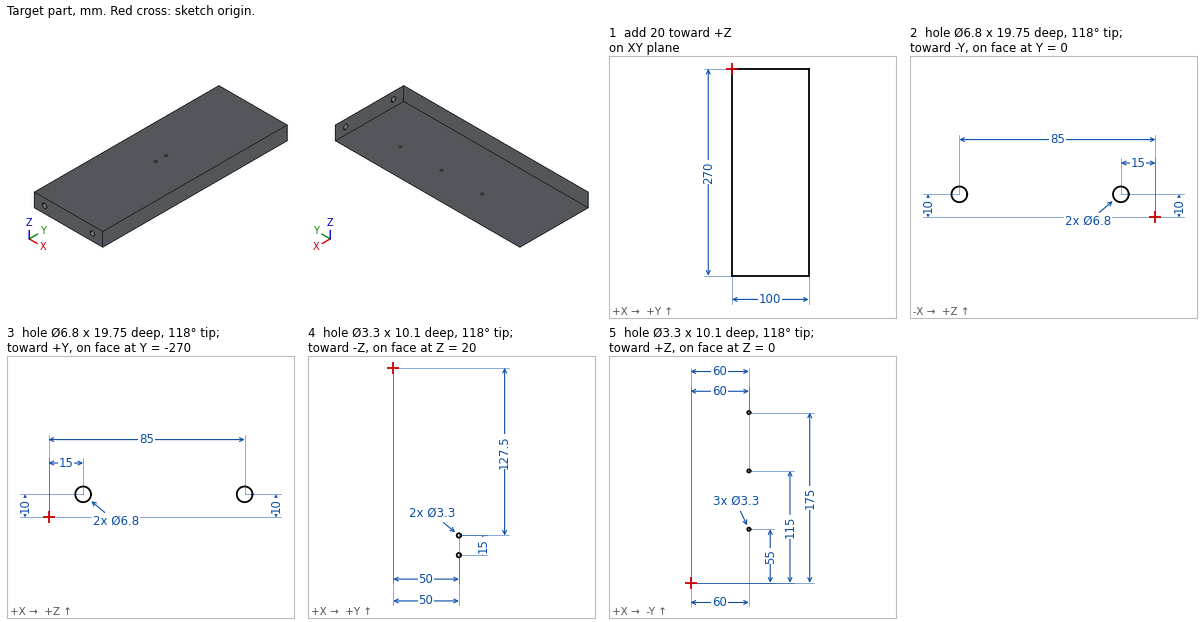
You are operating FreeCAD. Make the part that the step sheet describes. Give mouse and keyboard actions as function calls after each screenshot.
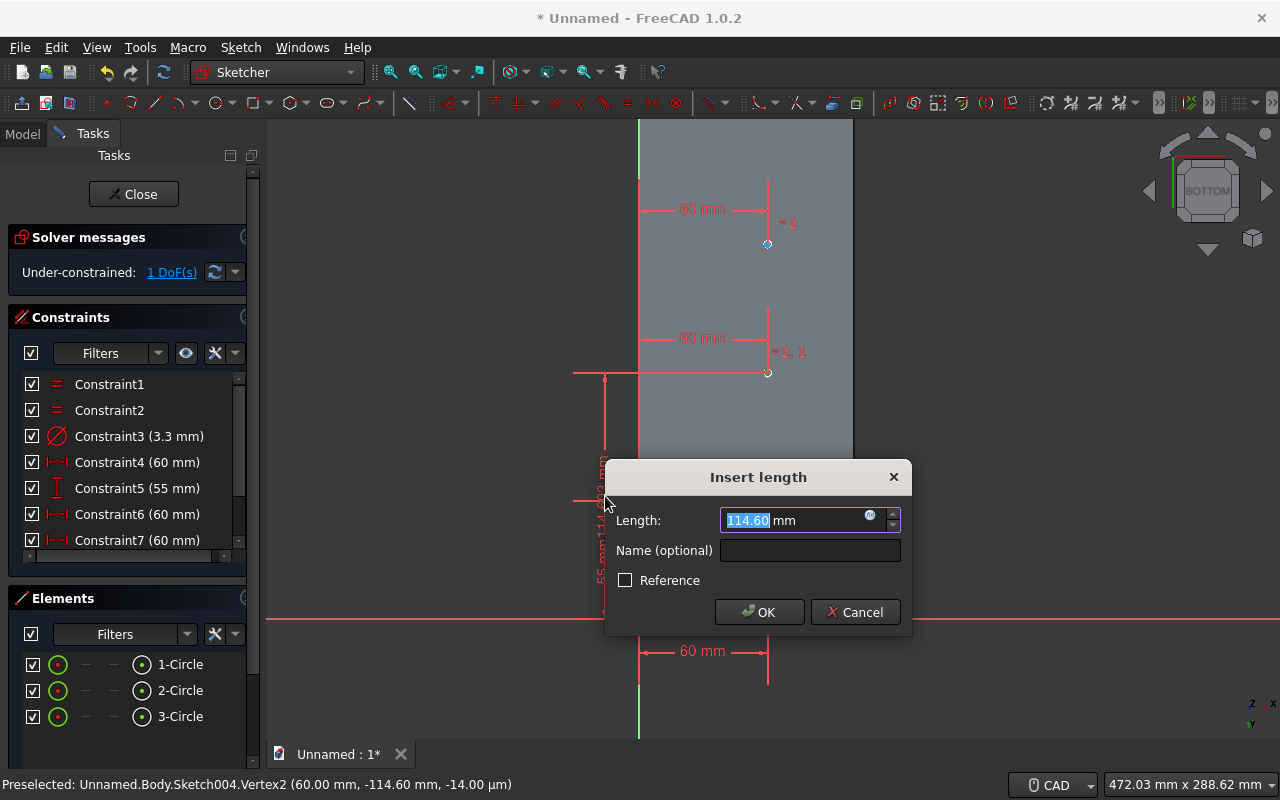
text(115)
key(Return)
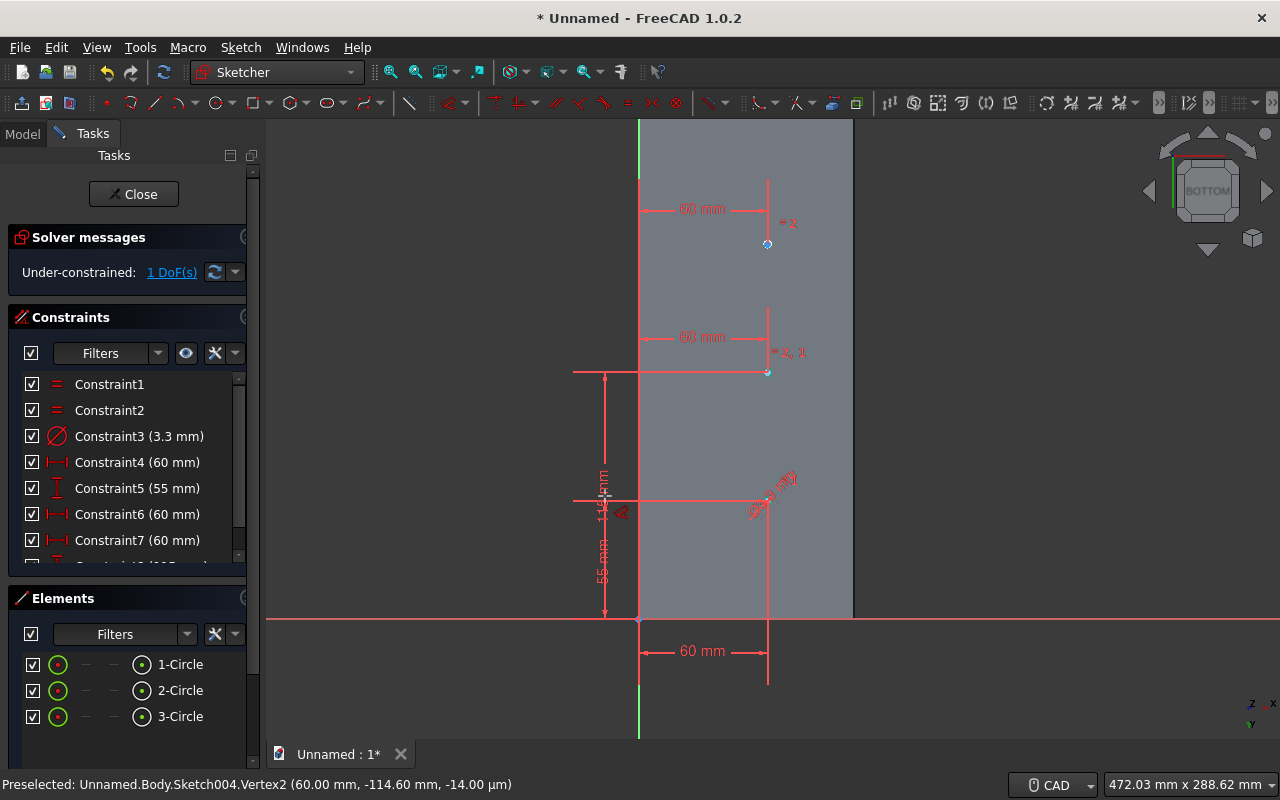
click(768, 244)
click(605, 432)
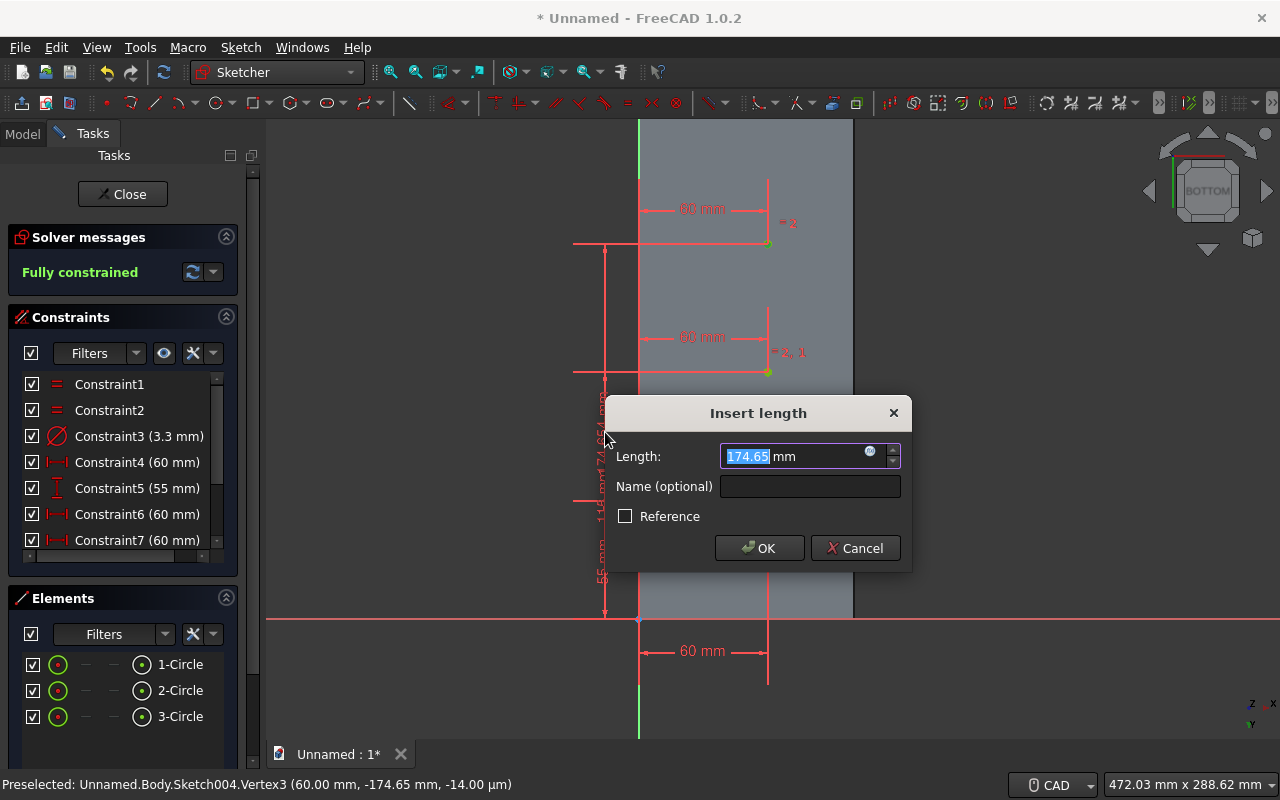
text(175)
key(Return)
key(Escape)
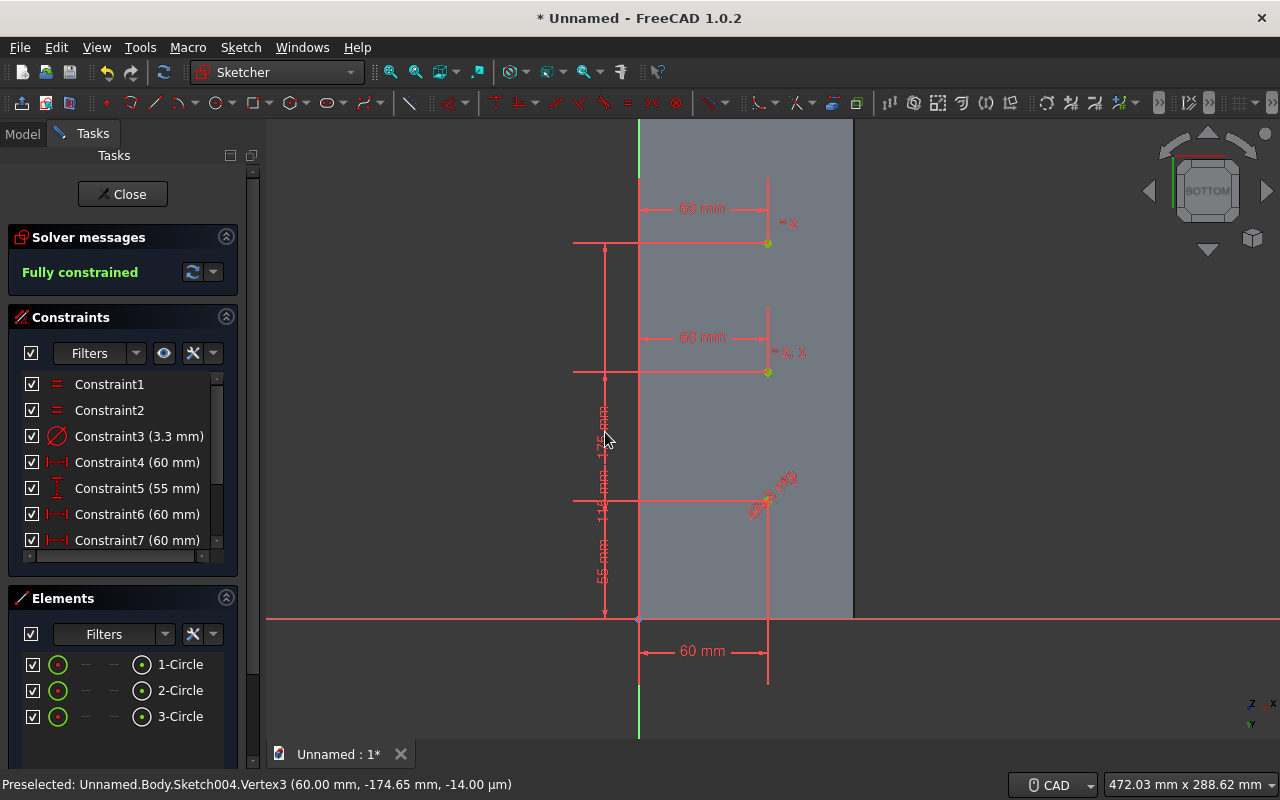
click(123, 194)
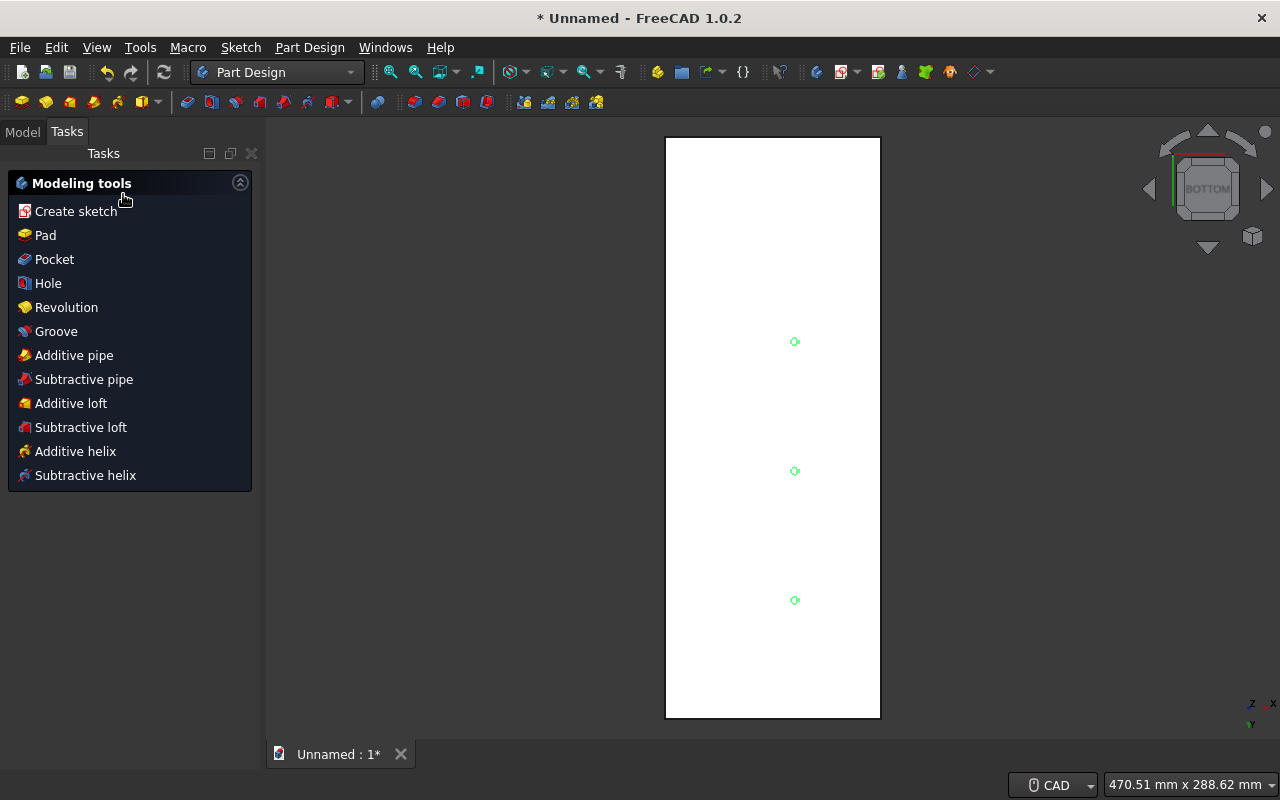
click(212, 102)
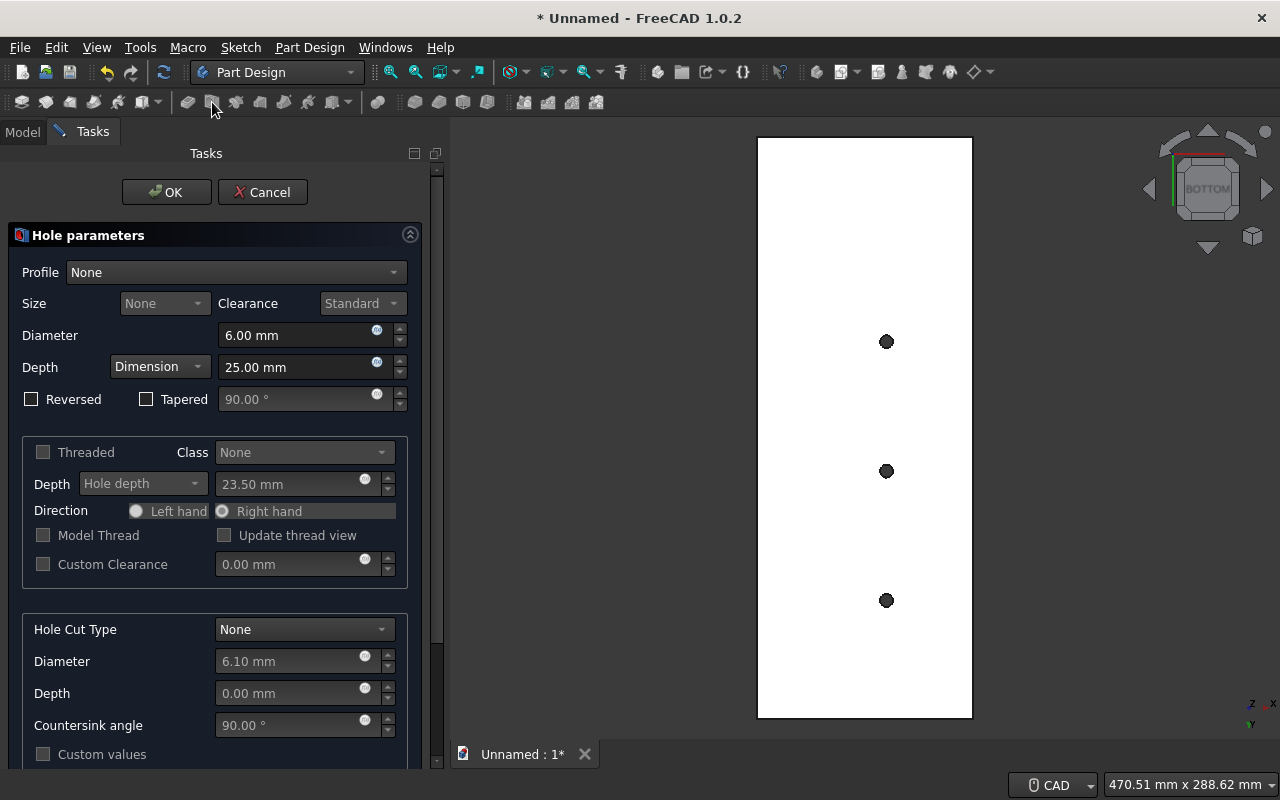
triple_click(305, 335)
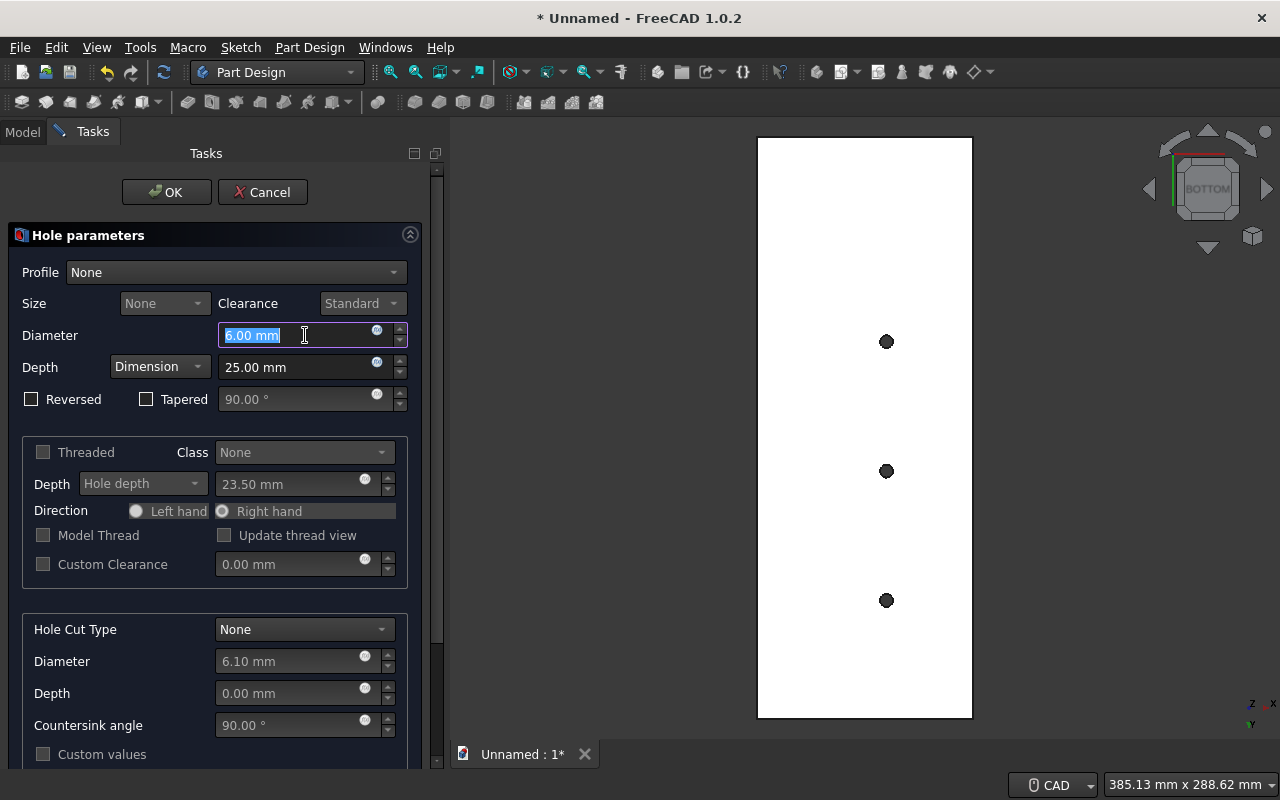
text(3.3)
key(Tab)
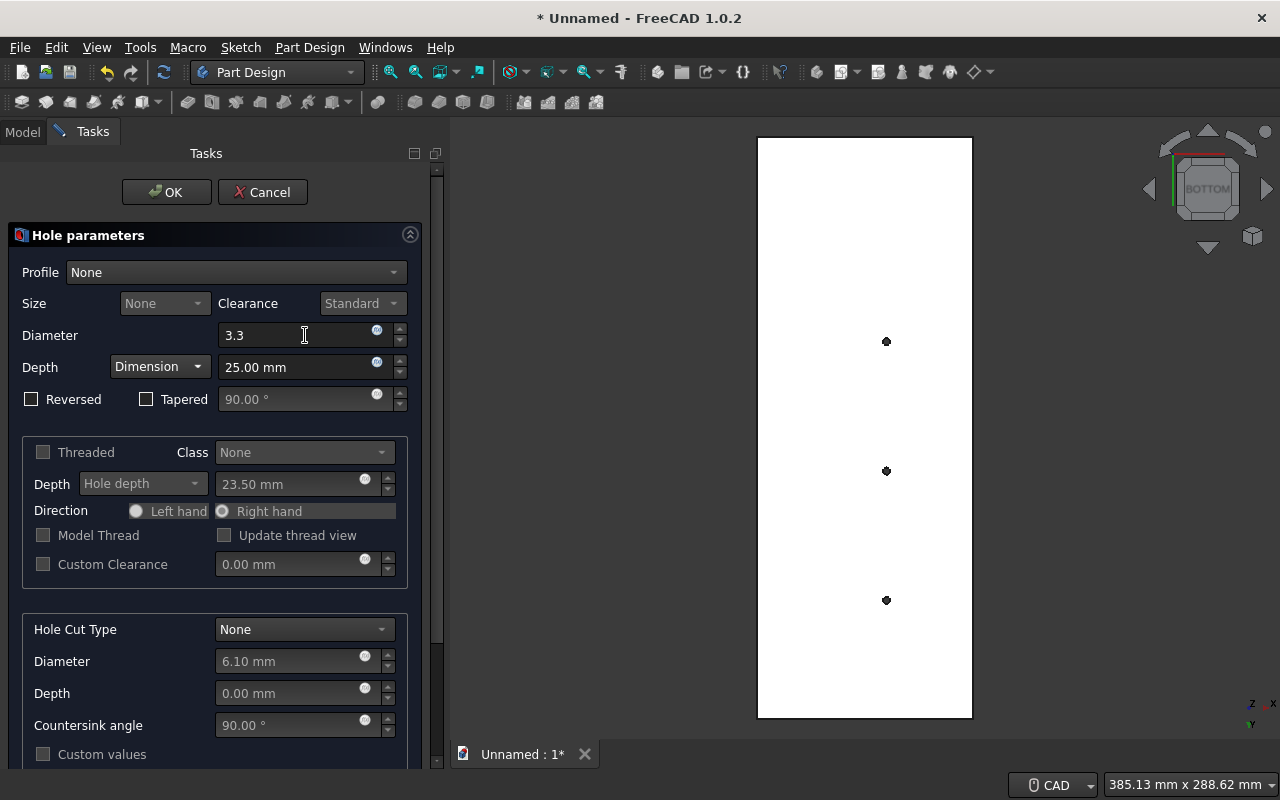
triple_click(305, 367)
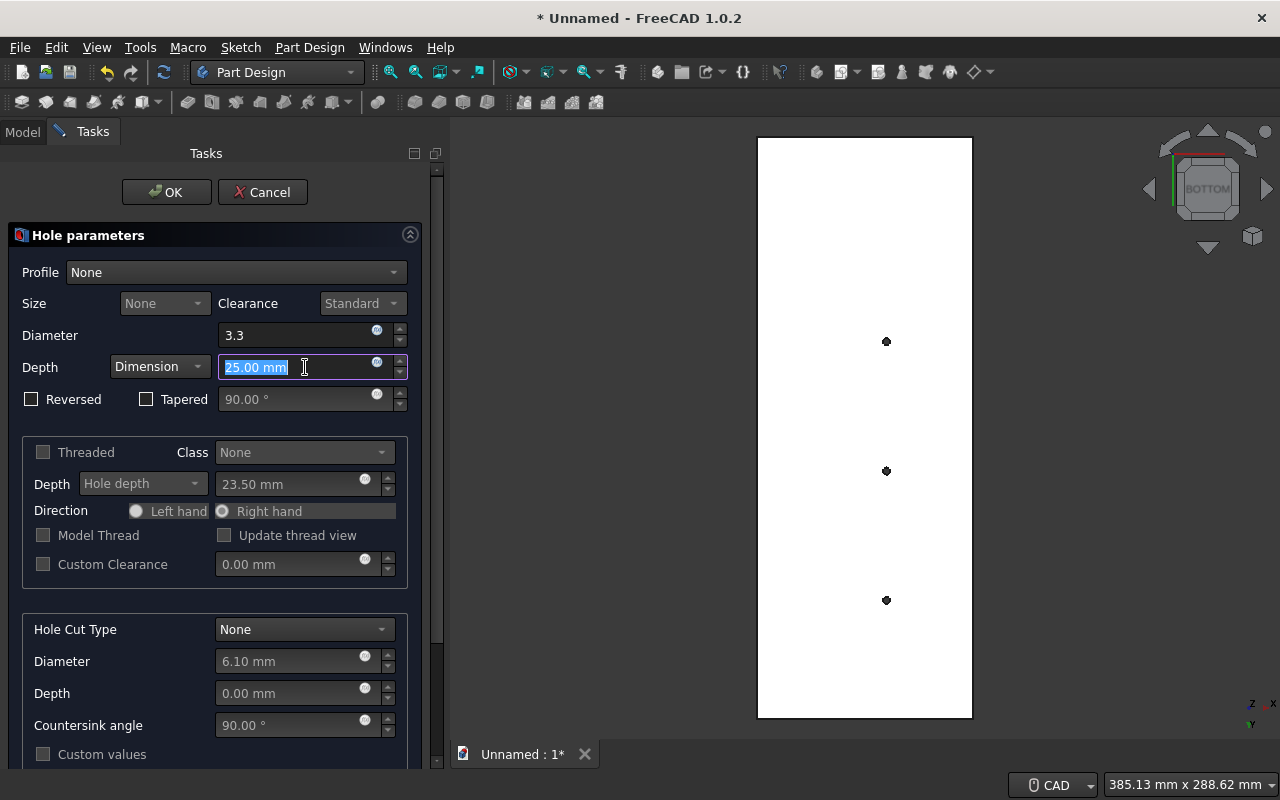
text(10.1)
key(Tab)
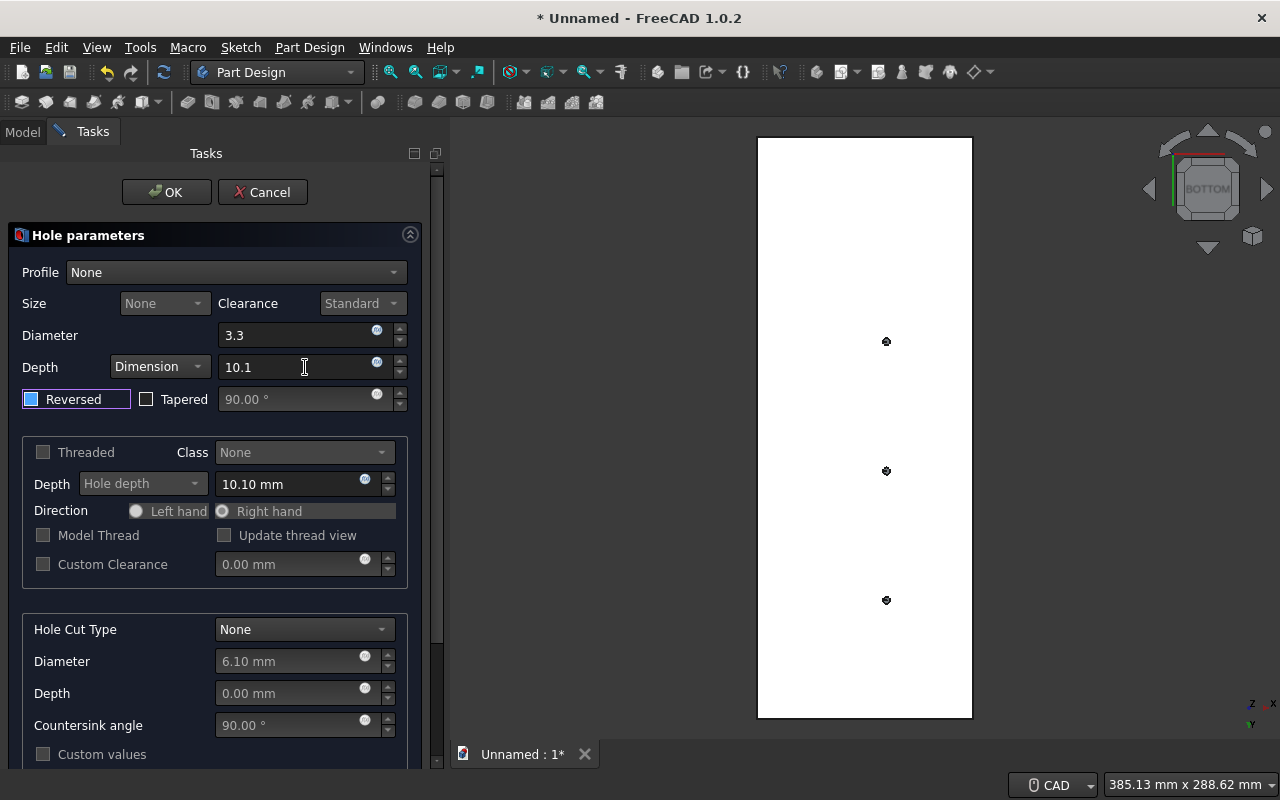
click(167, 192)